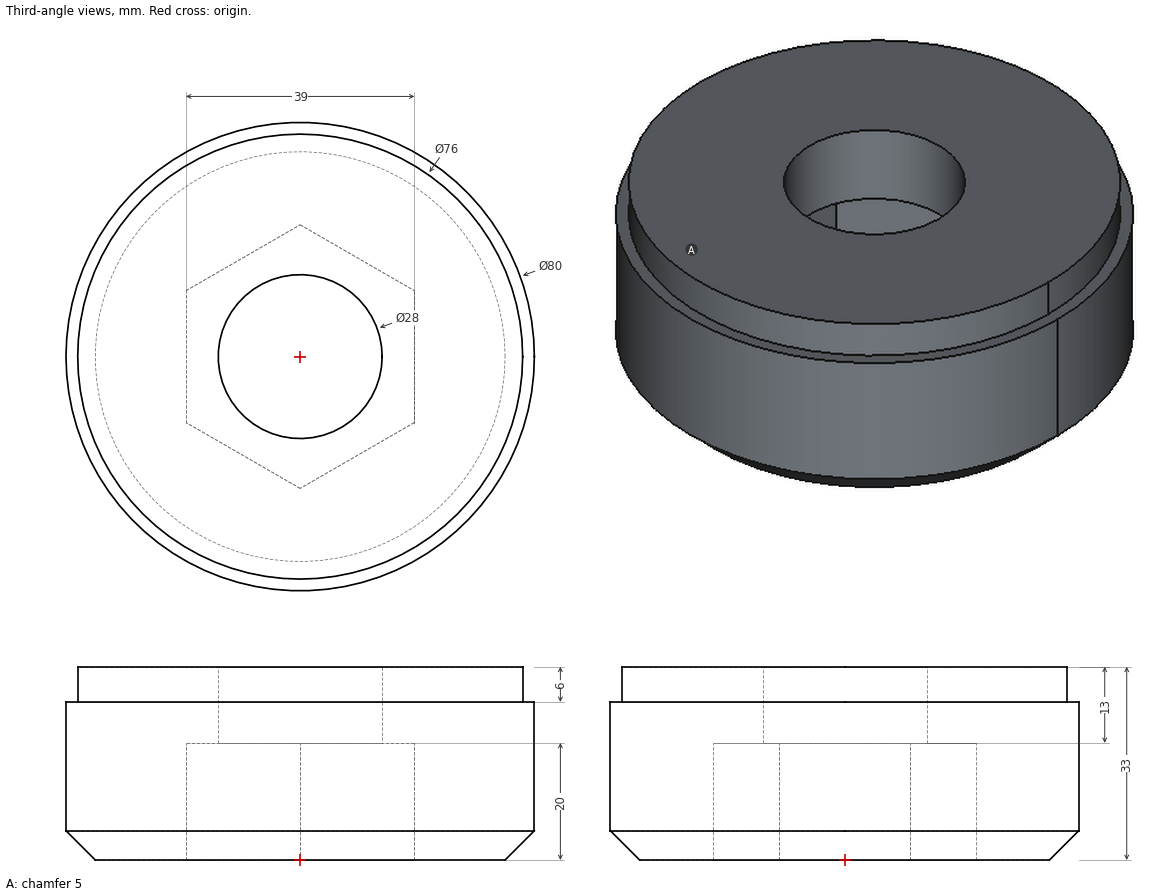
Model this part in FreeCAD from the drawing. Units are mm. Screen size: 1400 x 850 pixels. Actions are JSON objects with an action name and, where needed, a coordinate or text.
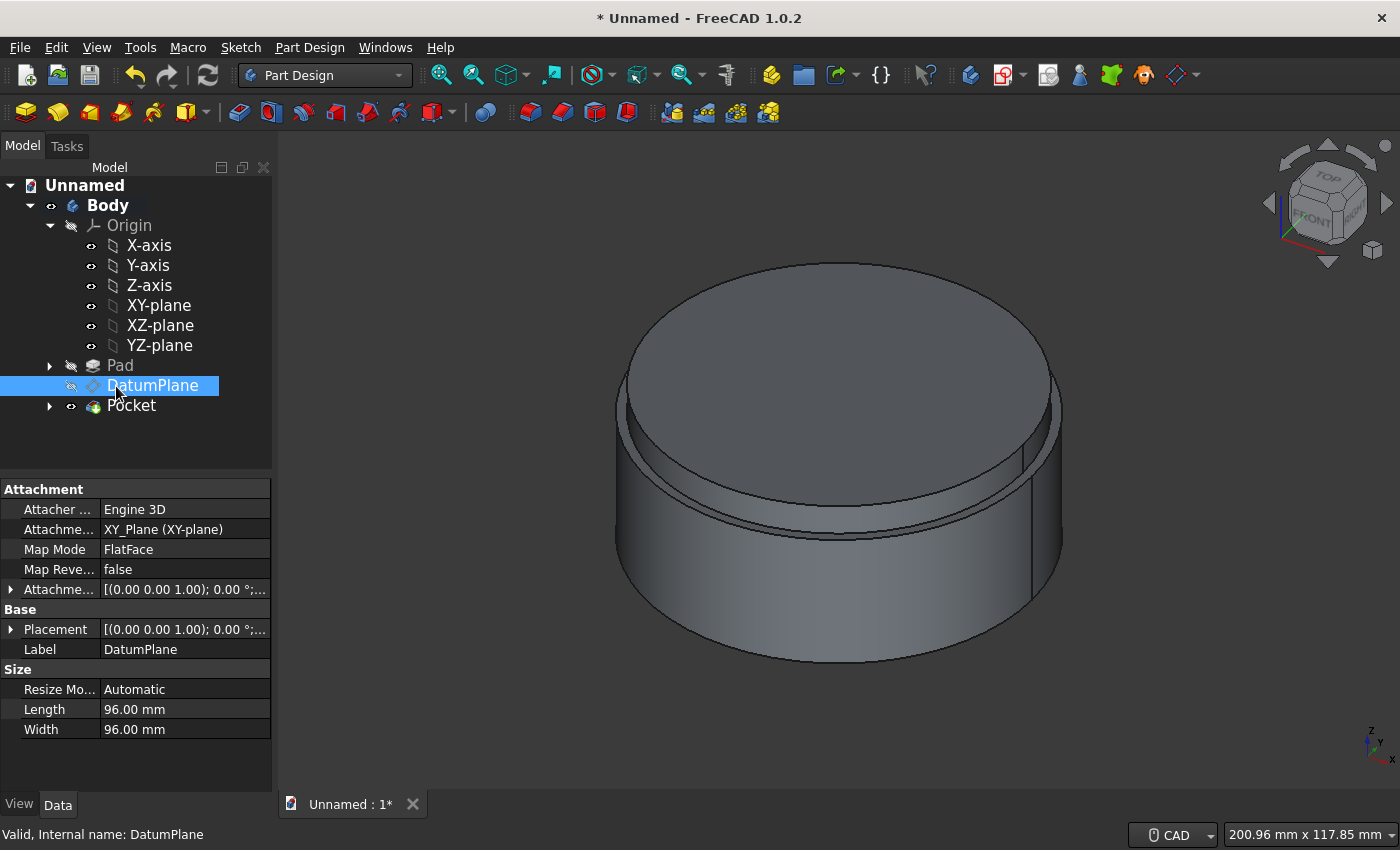
{"action": "key", "text": "0"}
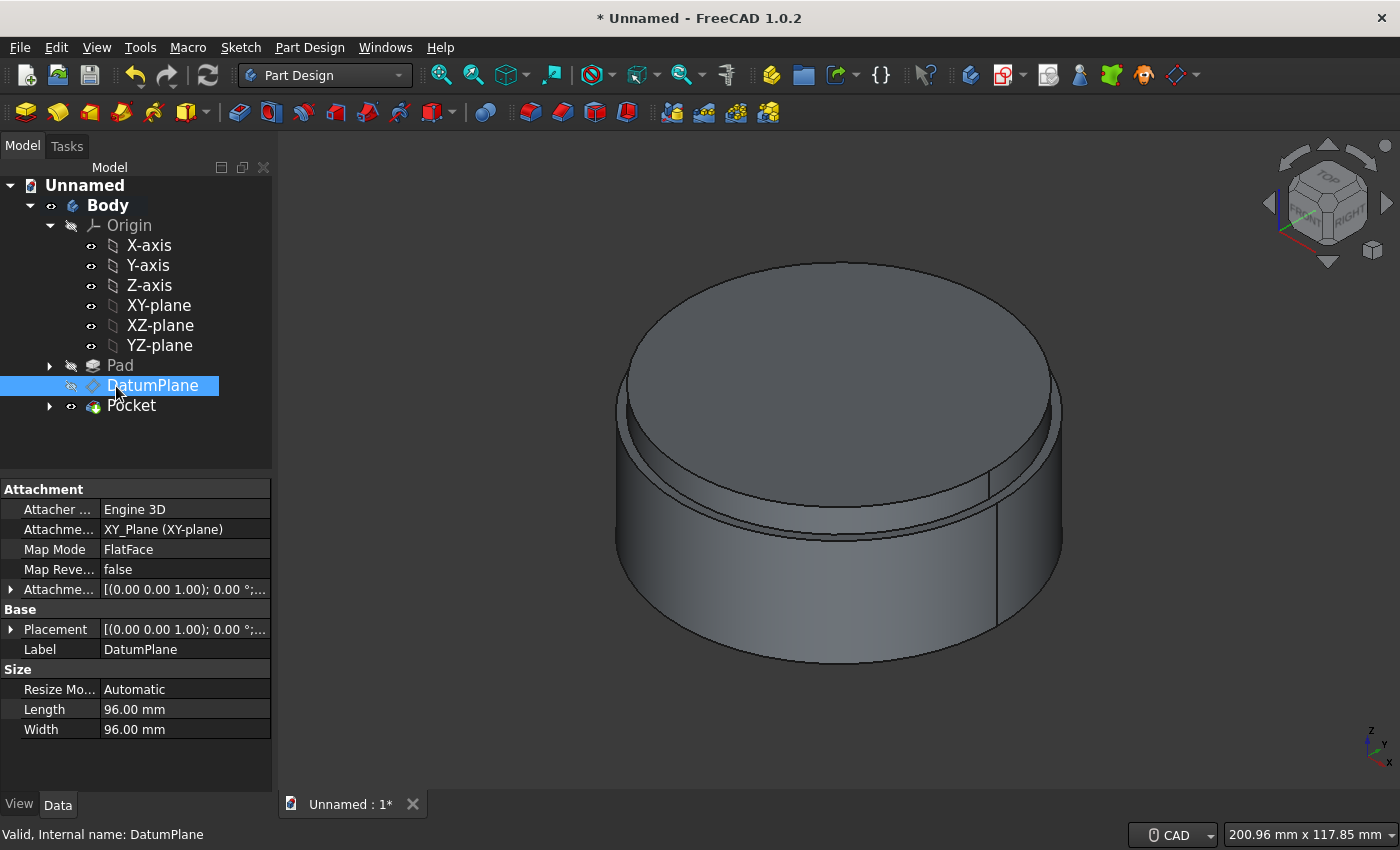
{"action": "key", "text": "2"}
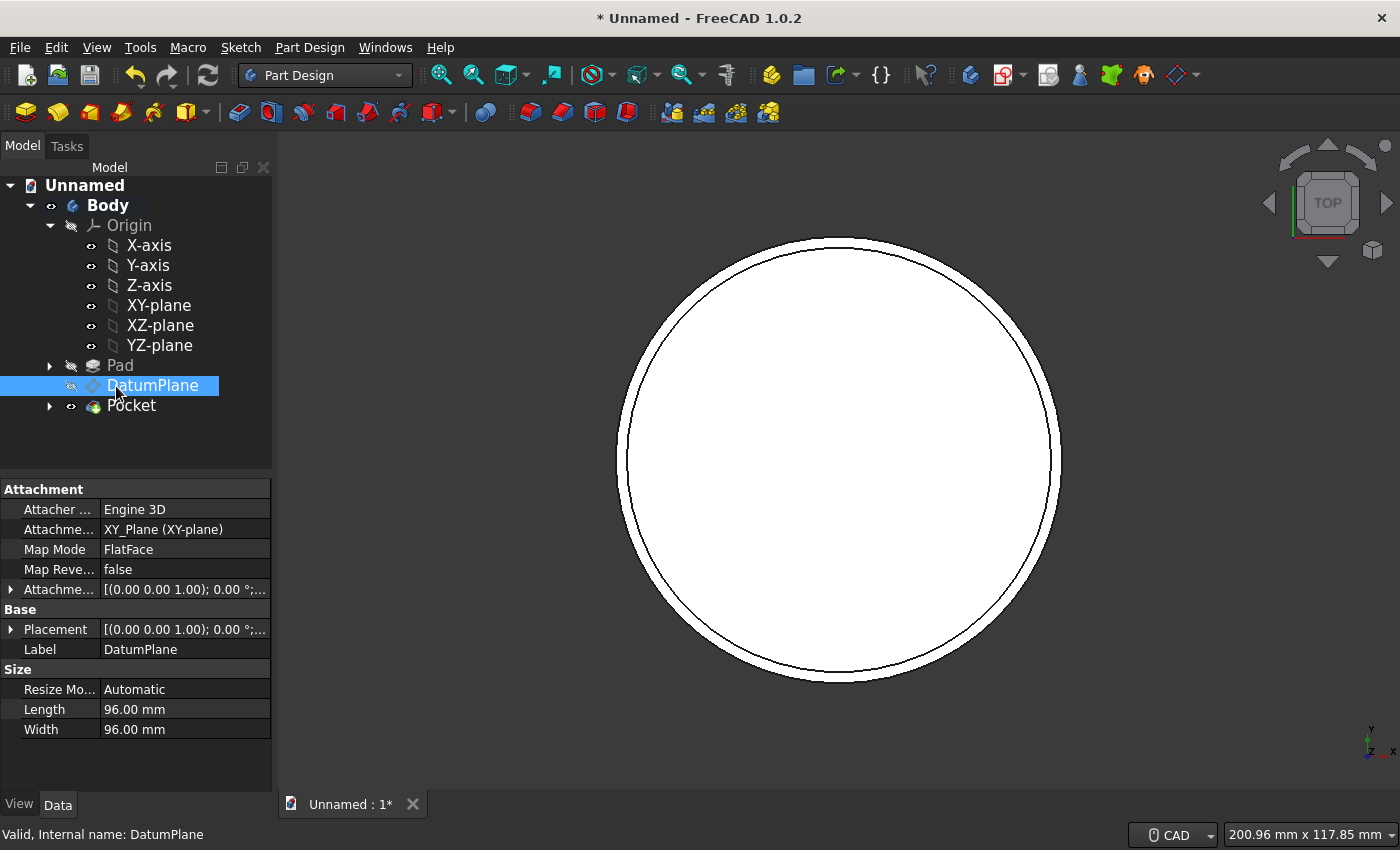
{"action": "key", "text": "1"}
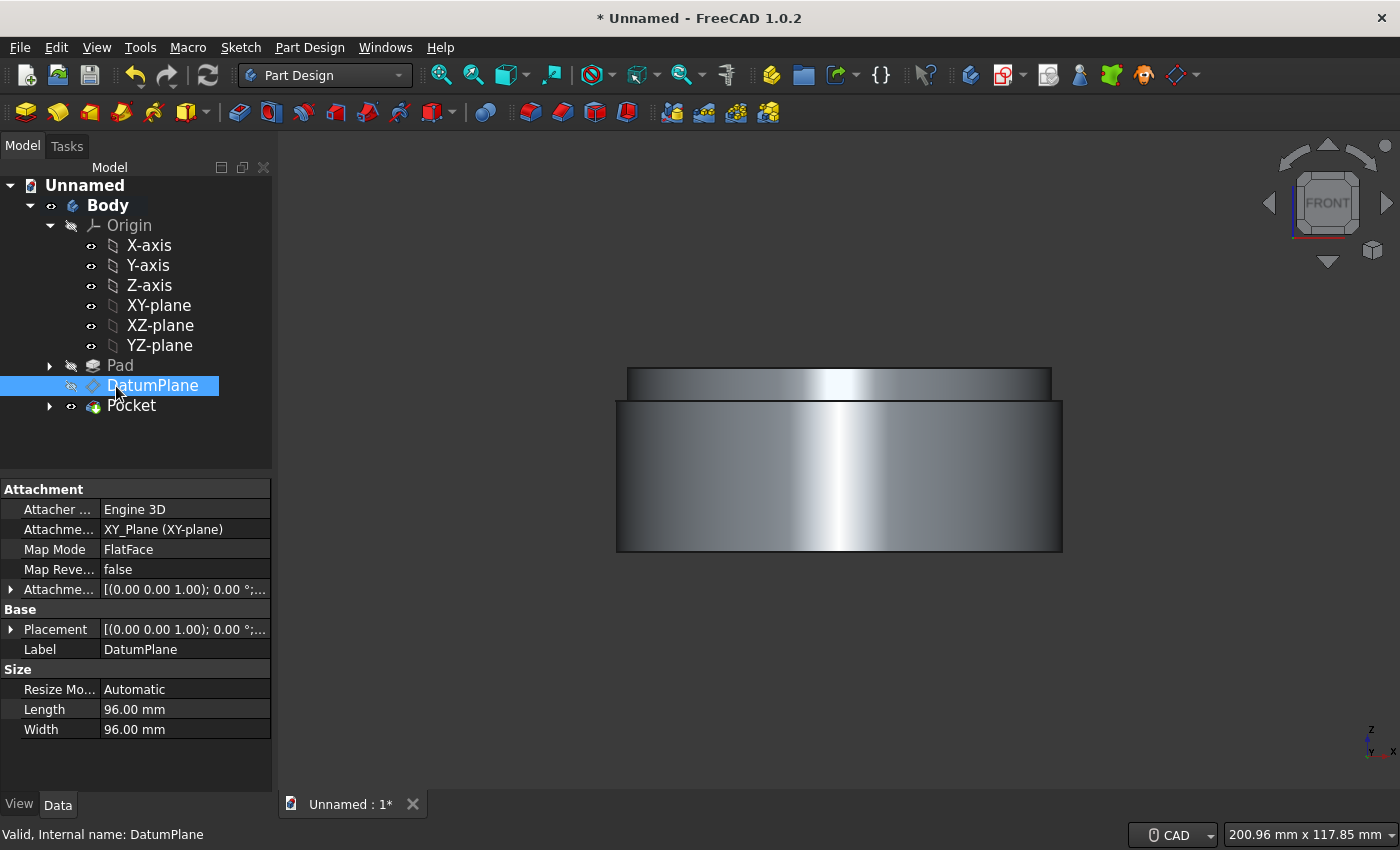
{"action": "left_click", "coordinate": [442, 76]}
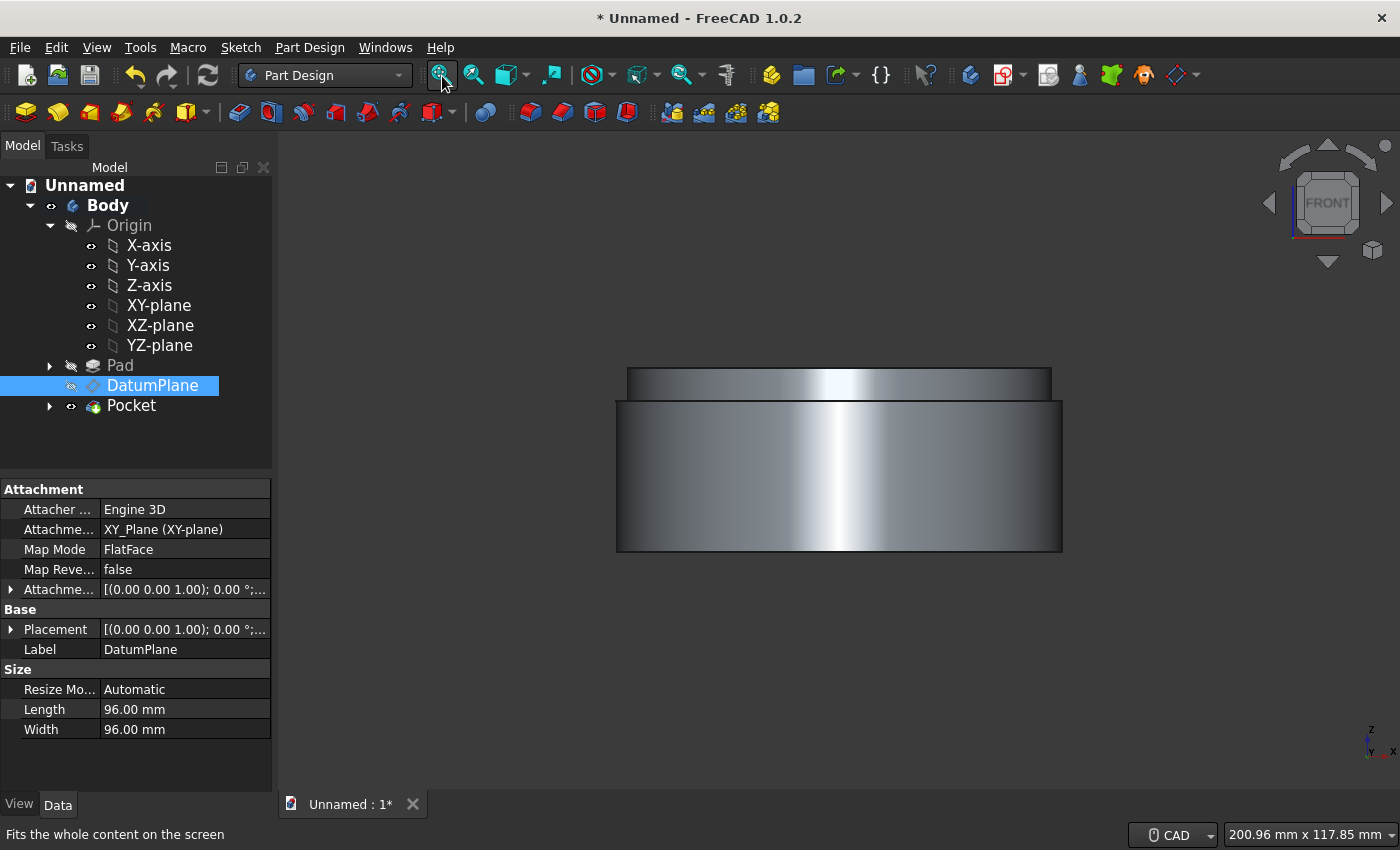
{"action": "left_click", "coordinate": [658, 551]}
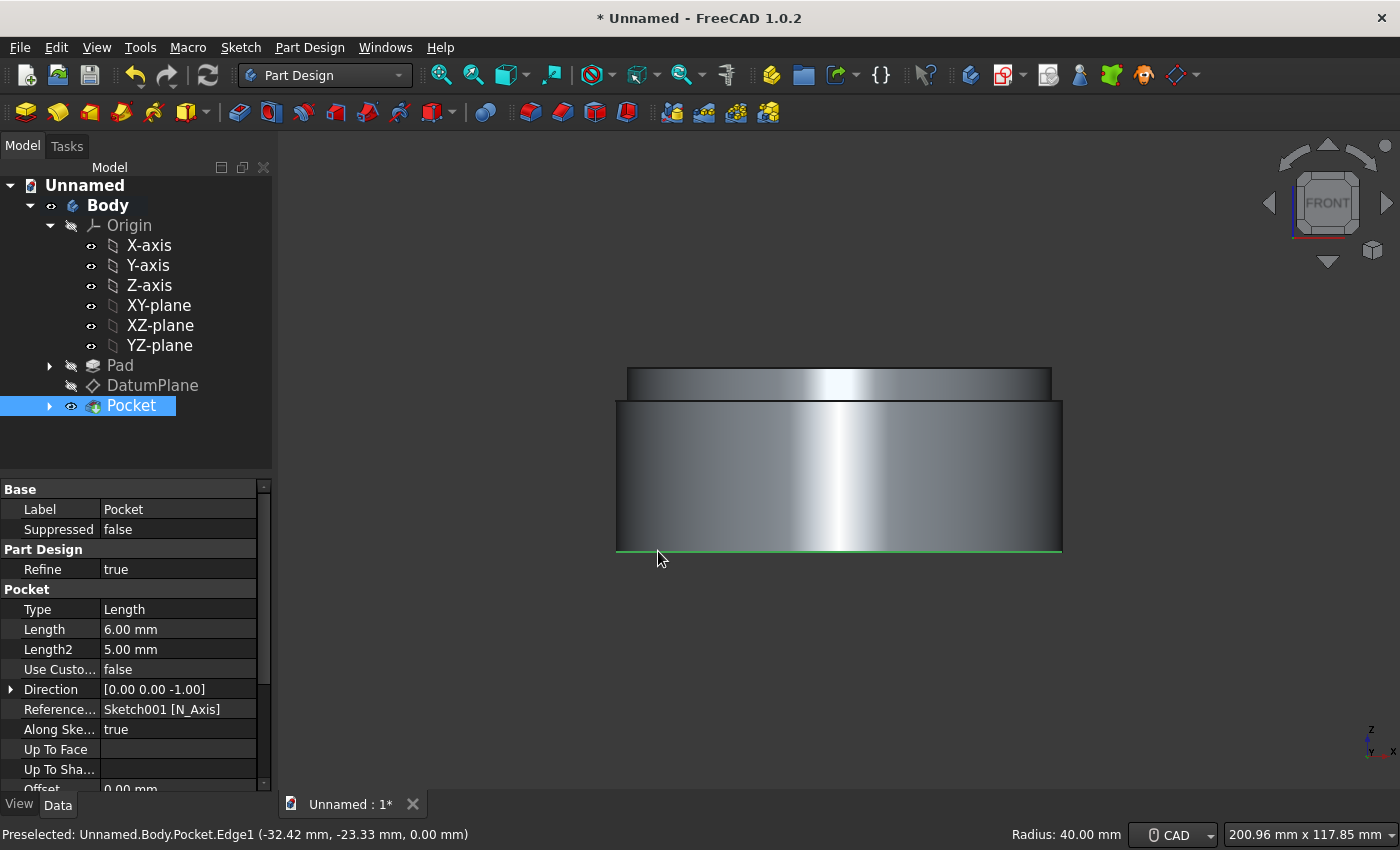
{"action": "left_click", "coordinate": [564, 112]}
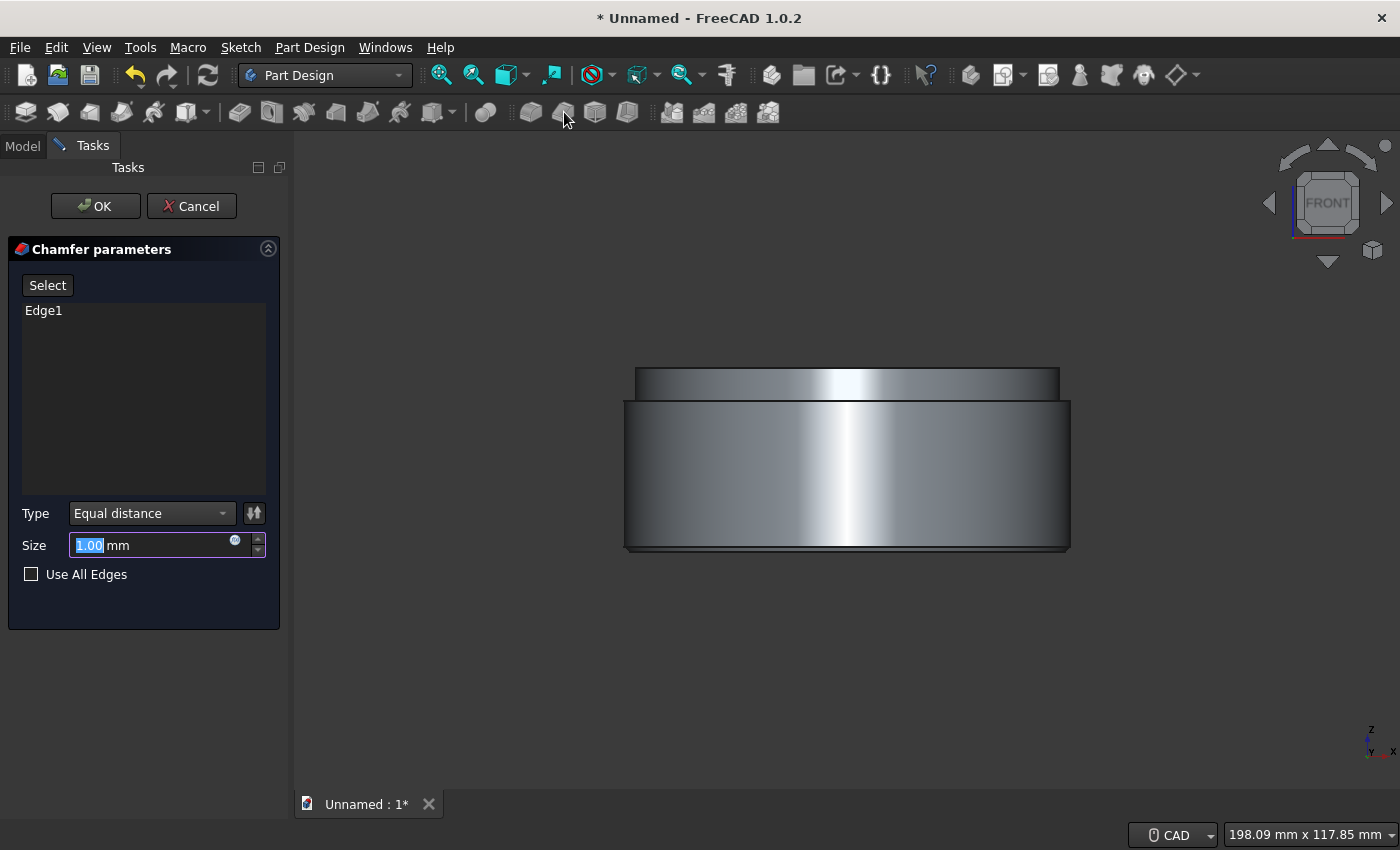
{"action": "type", "text": "5"}
{"action": "key", "text": "Tab"}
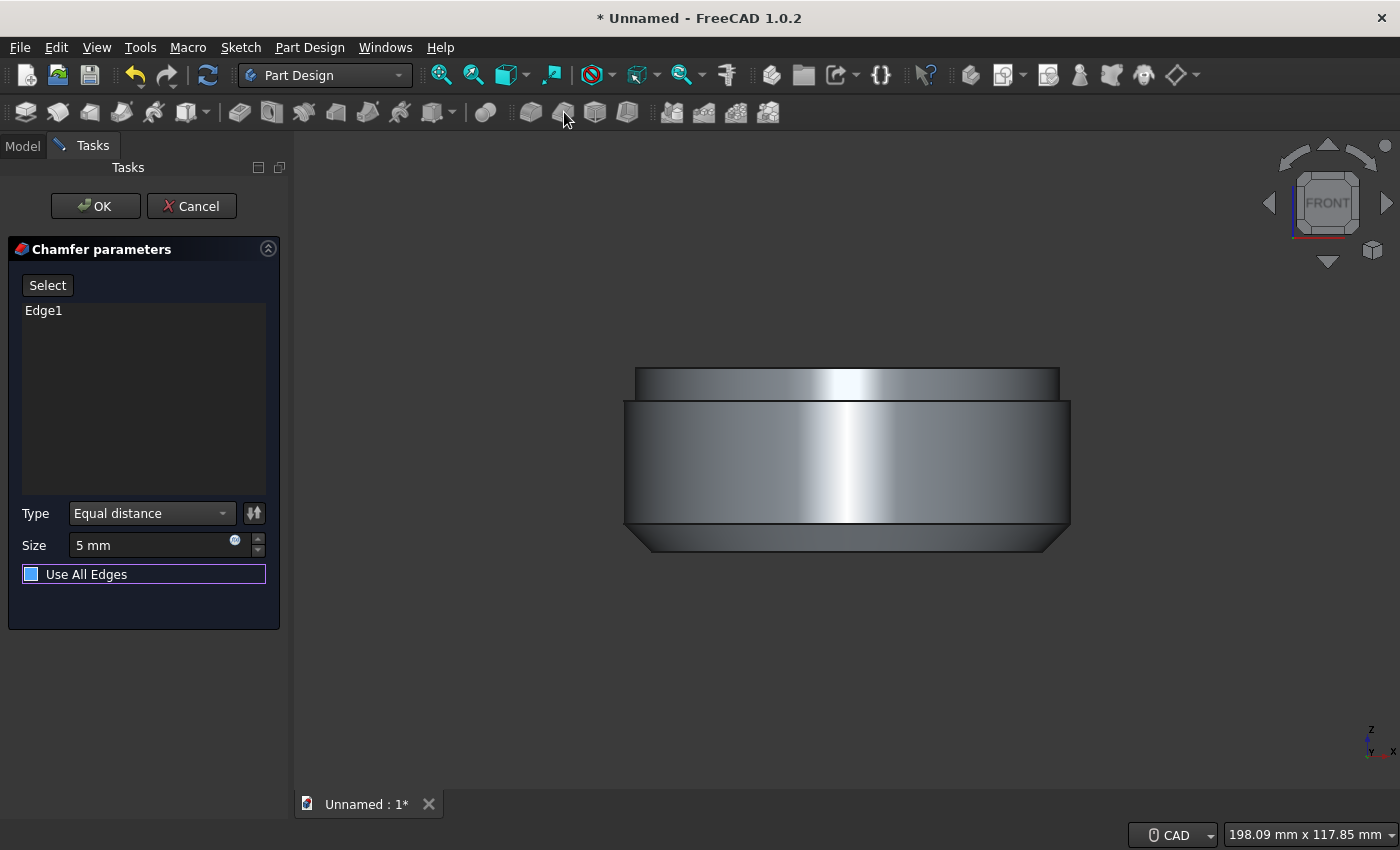
{"action": "left_click", "coordinate": [96, 206]}